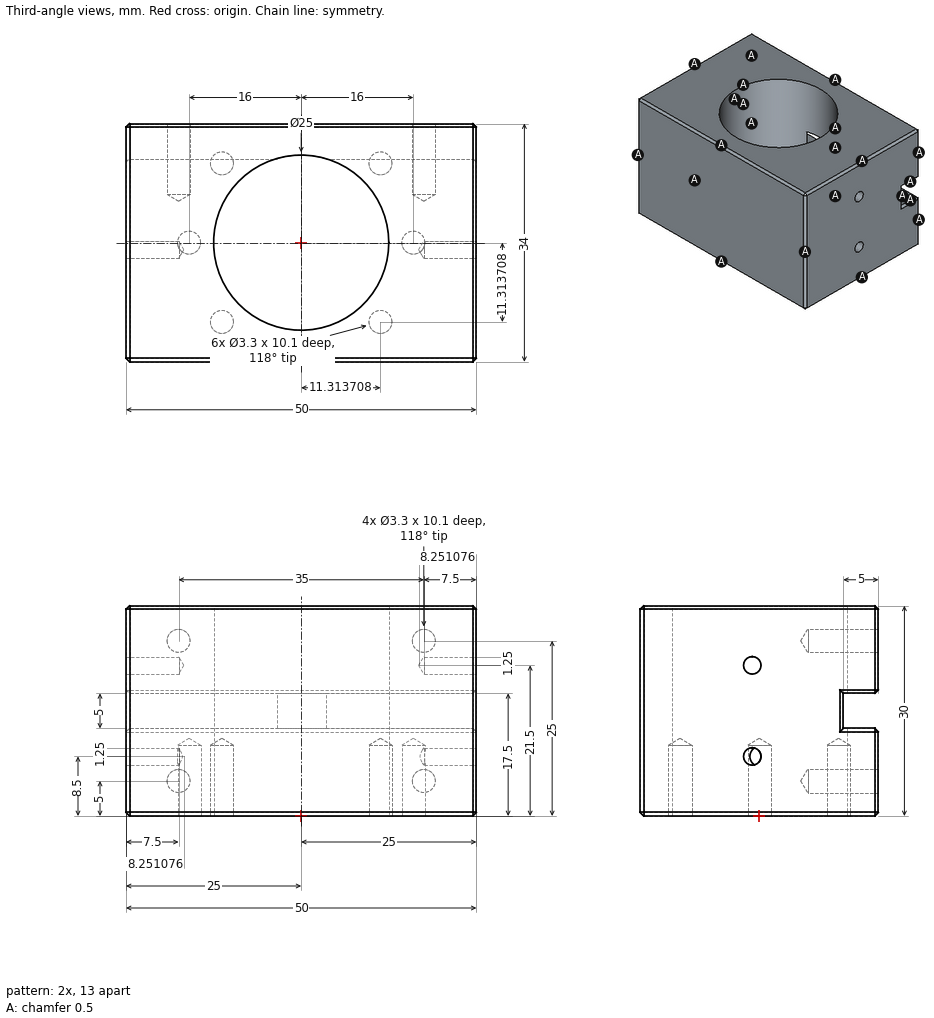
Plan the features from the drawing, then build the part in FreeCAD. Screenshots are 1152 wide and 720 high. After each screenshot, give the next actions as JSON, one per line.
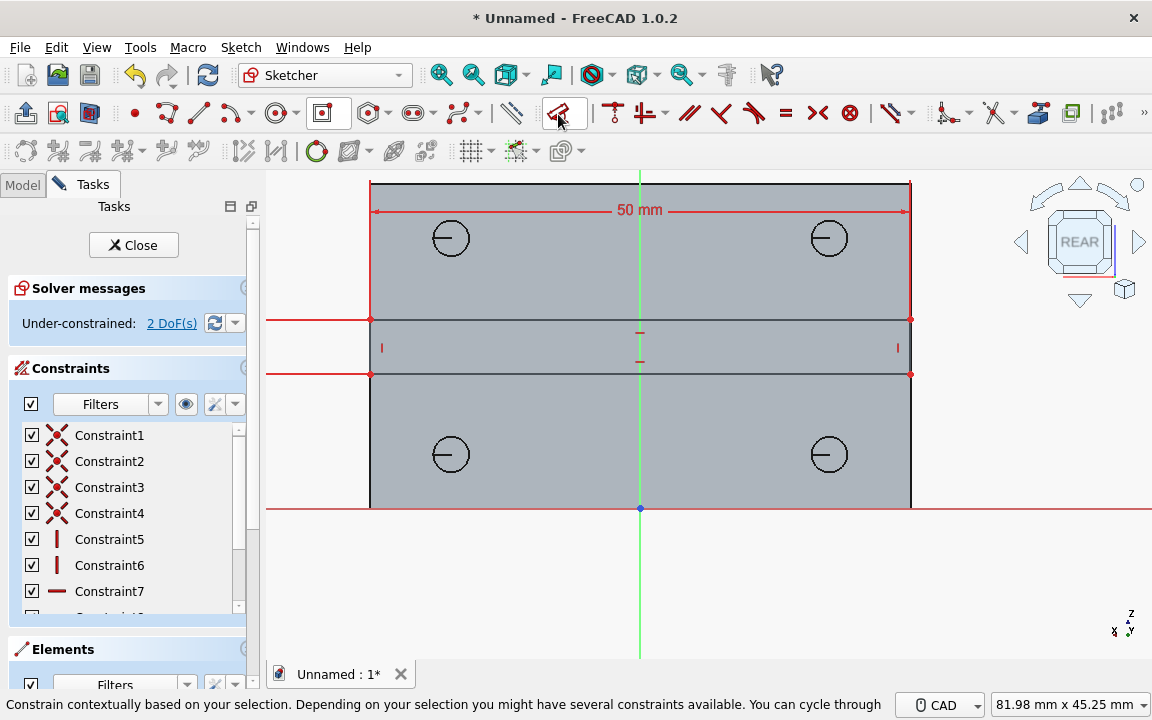
{"action": "left_click", "coordinate": [370, 320]}
{"action": "left_click", "coordinate": [505, 543]}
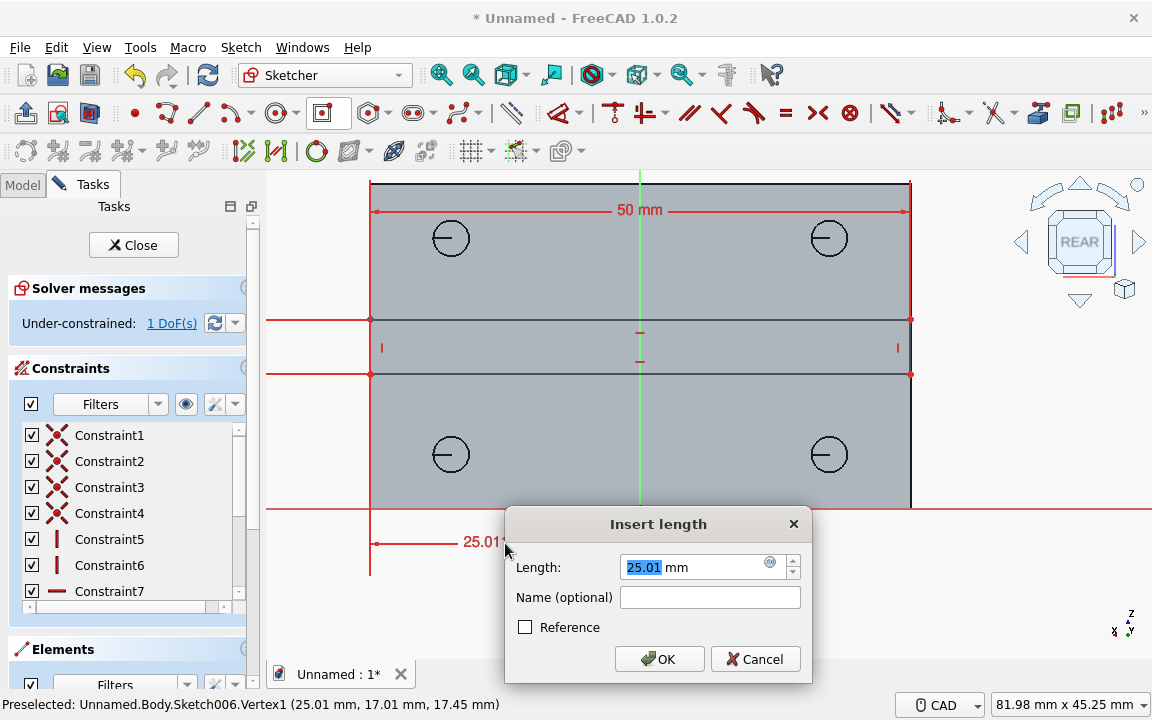
{"action": "type", "text": "25"}
{"action": "key", "text": "Return"}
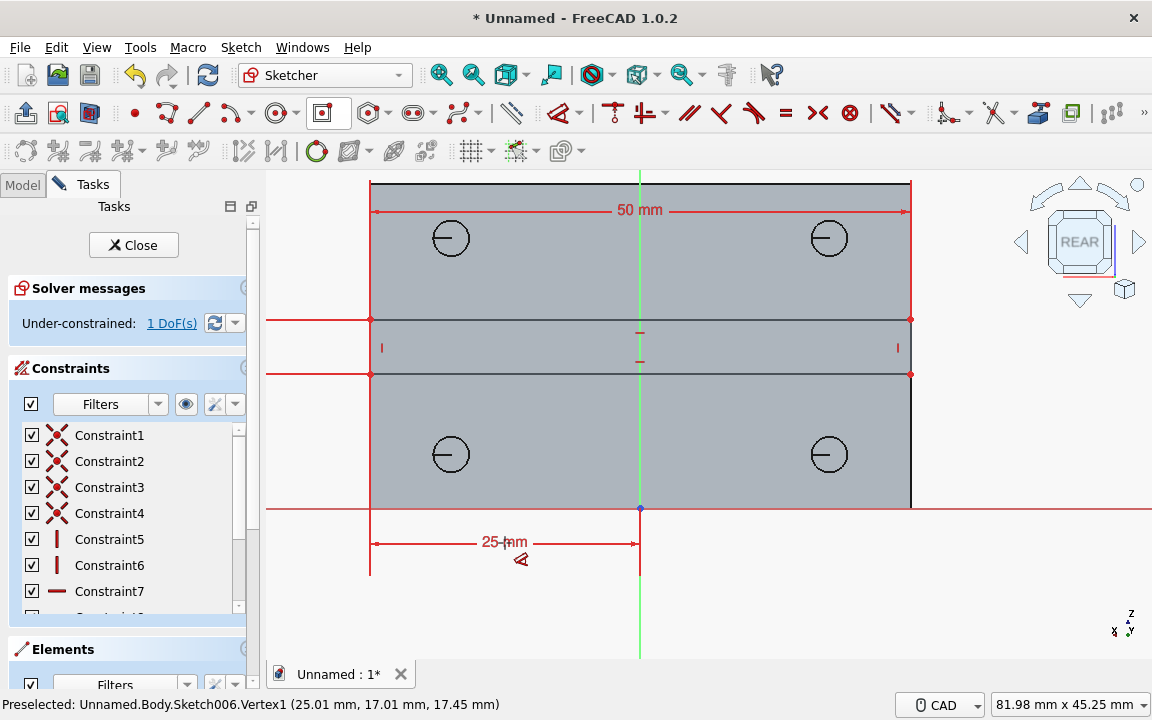
{"action": "left_click", "coordinate": [370, 320]}
{"action": "left_click", "coordinate": [336, 414]}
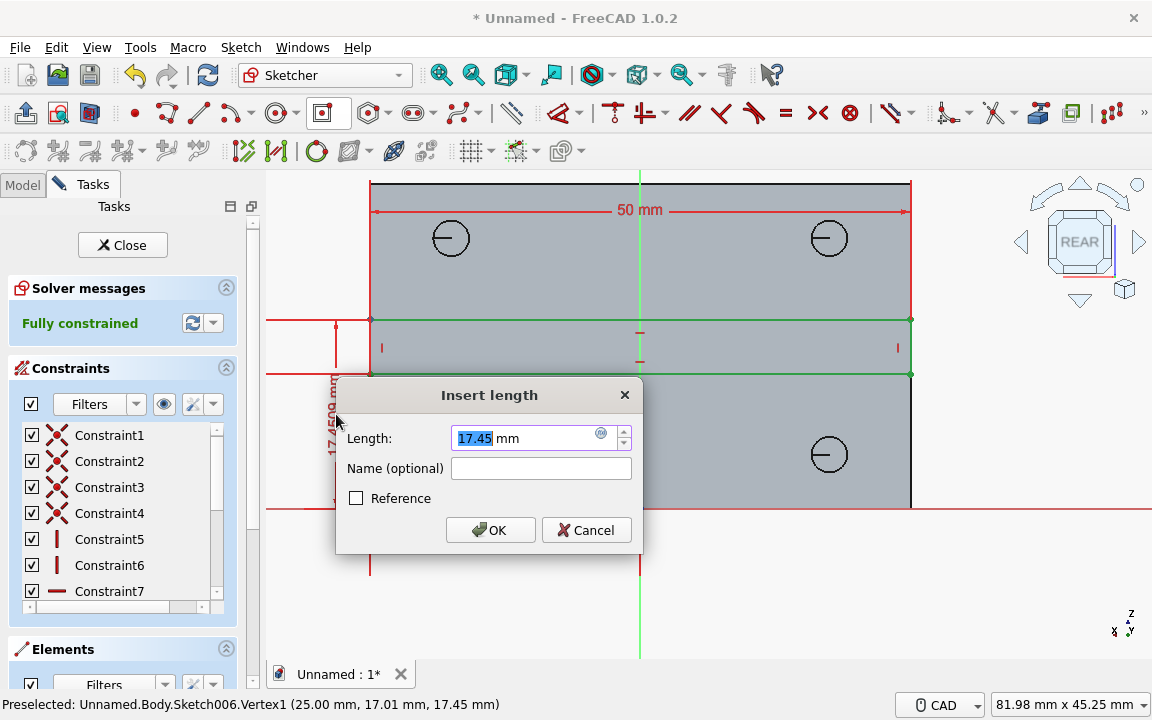
{"action": "type", "text": "17.5"}
{"action": "key", "text": "Return"}
{"action": "key", "text": "Escape"}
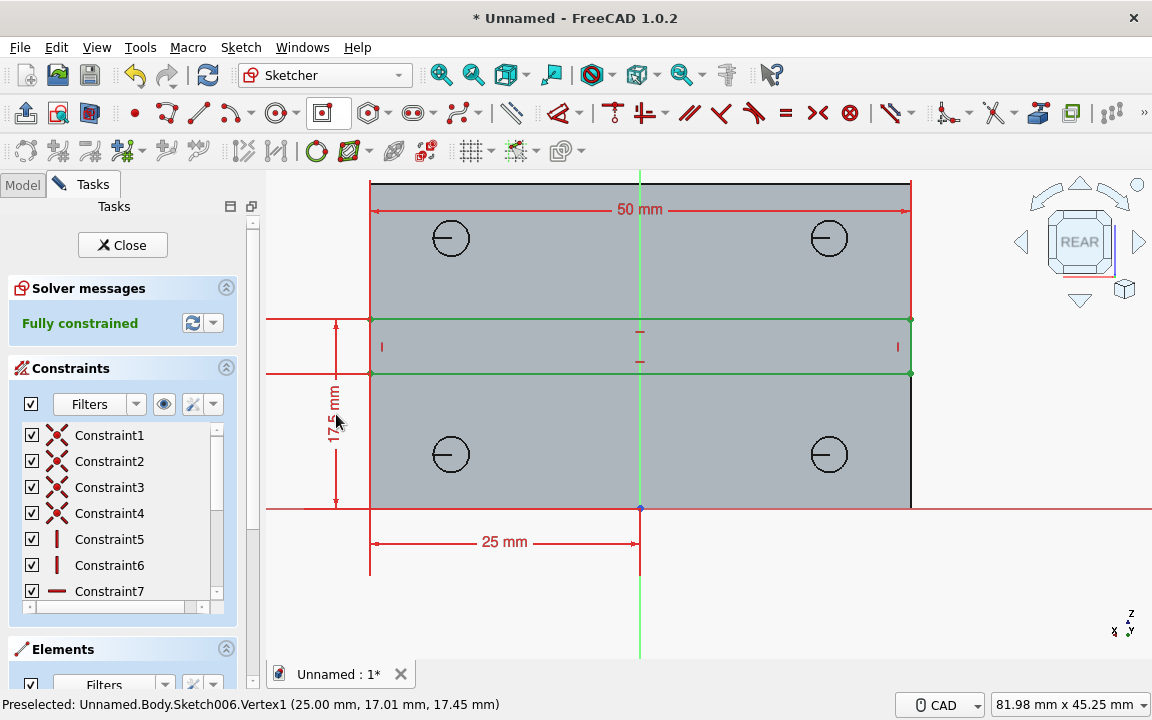
{"action": "left_click", "coordinate": [123, 245]}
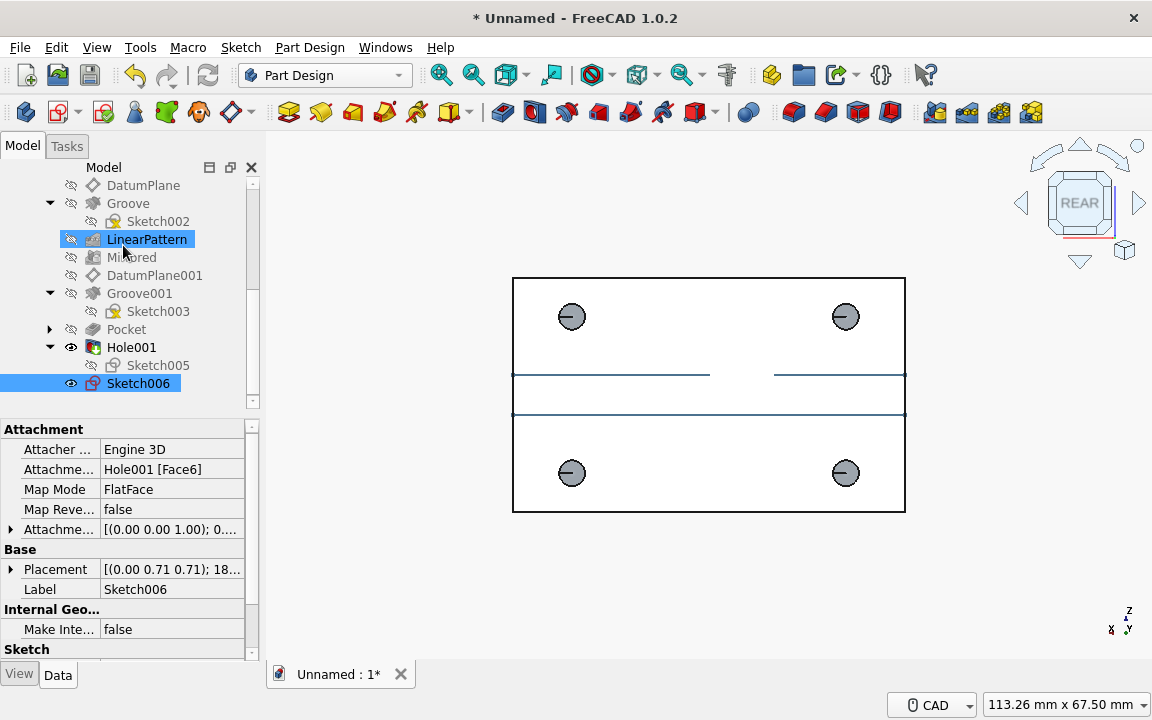
{"action": "left_click", "coordinate": [504, 112]}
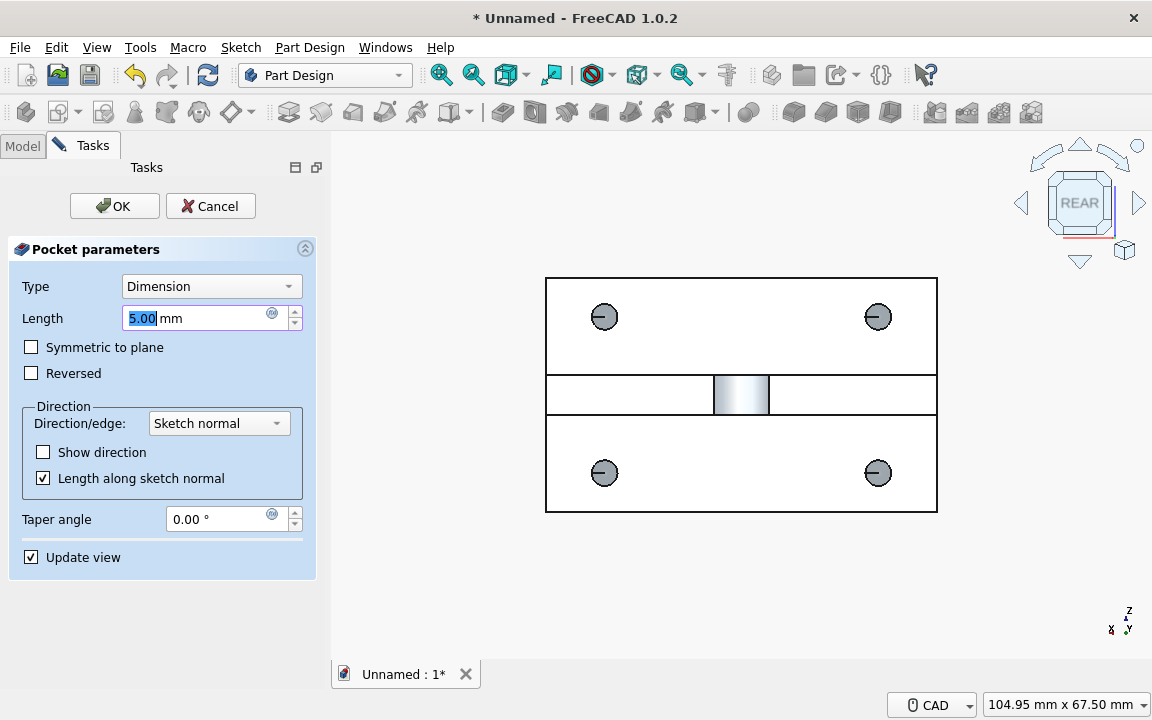
{"action": "type", "text": "5"}
{"action": "key", "text": "Tab"}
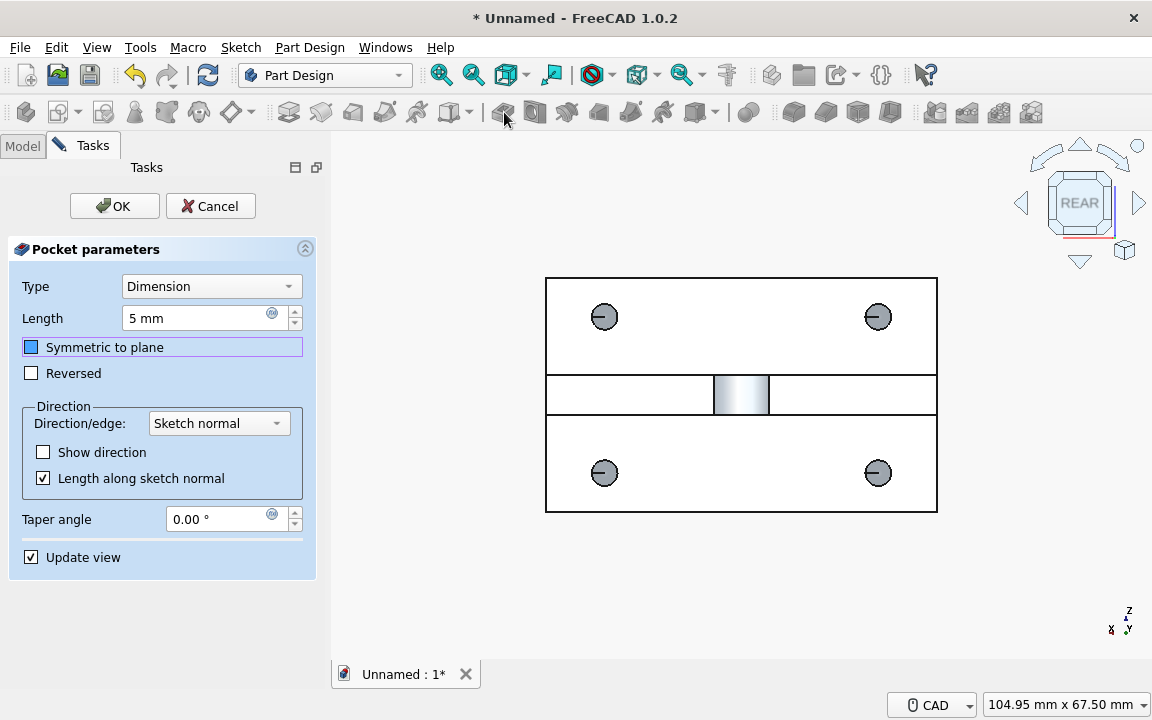
{"action": "left_click", "coordinate": [115, 206]}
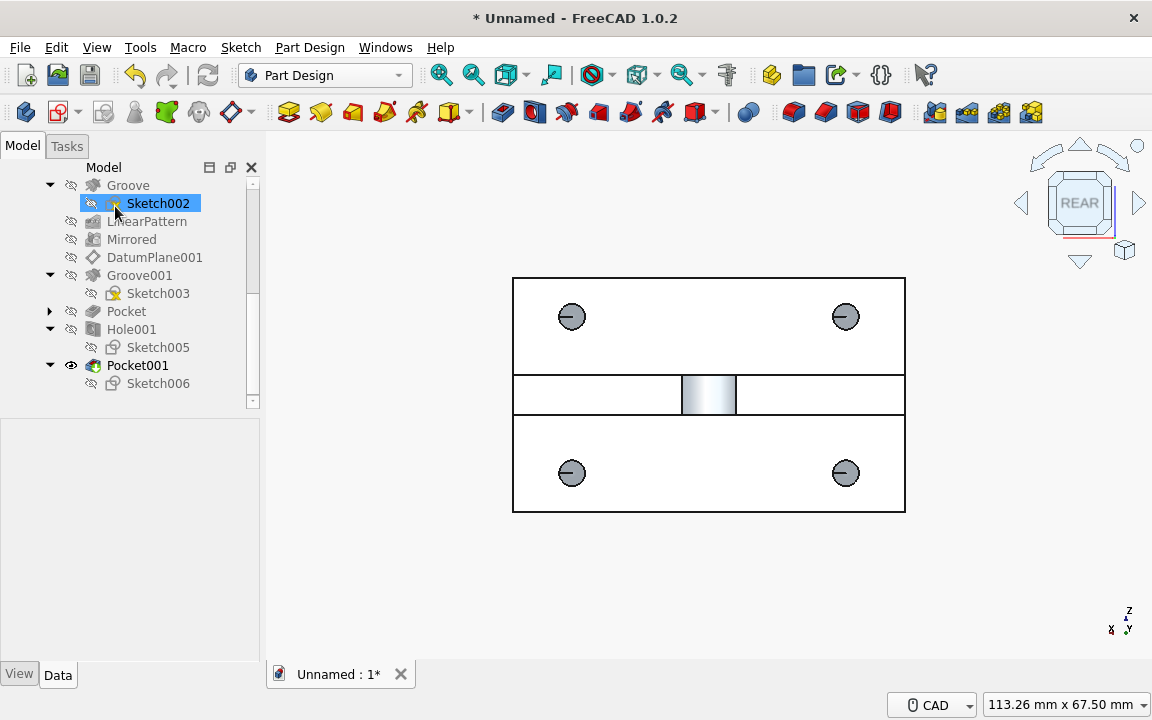
{"action": "key", "text": "v f"}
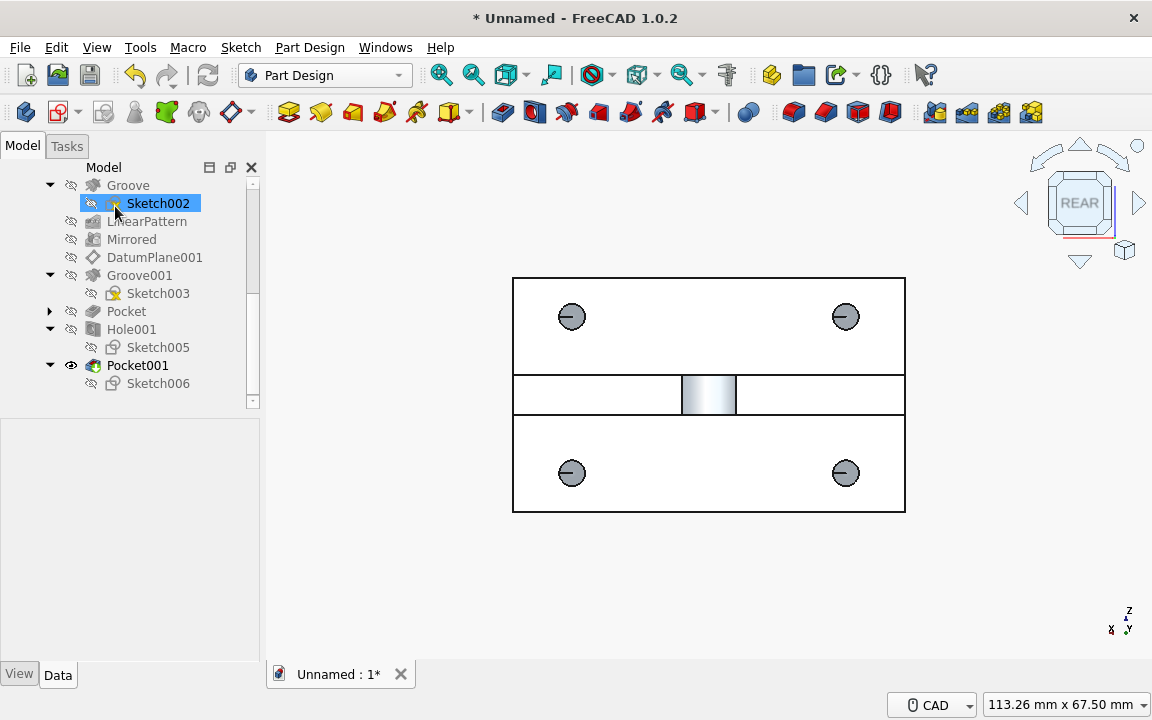
{"action": "left_click", "coordinate": [709, 374]}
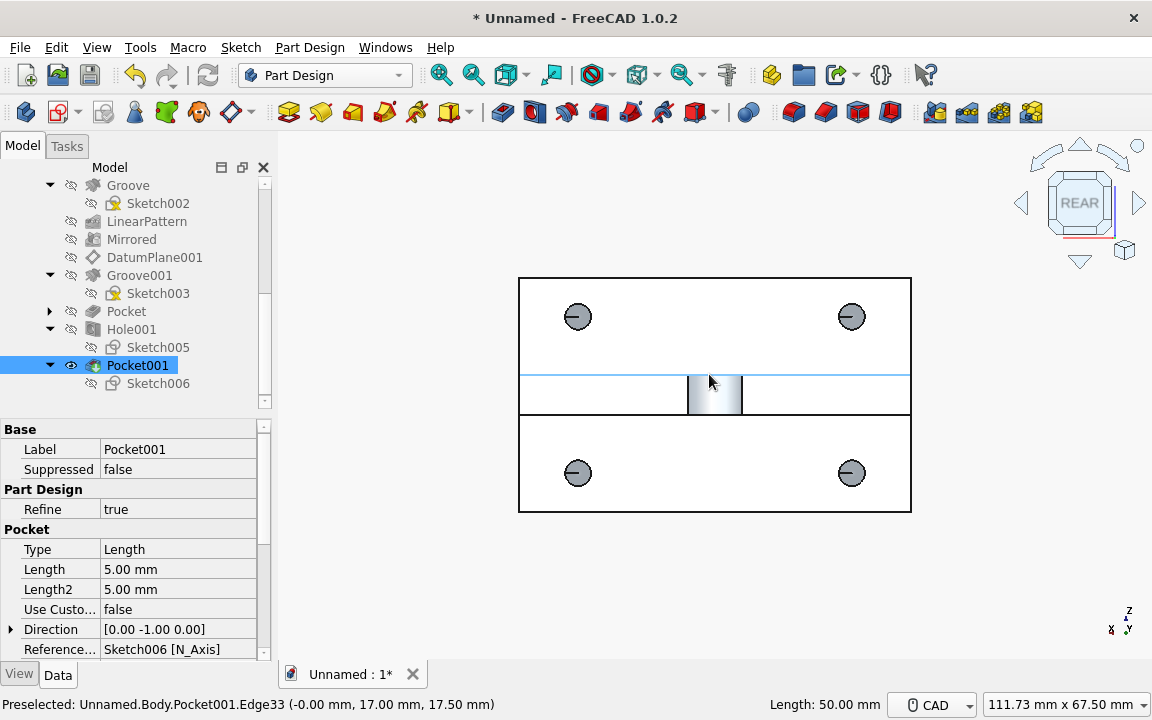
{"action": "left_click", "coordinate": [715, 511], "text": "ctrl"}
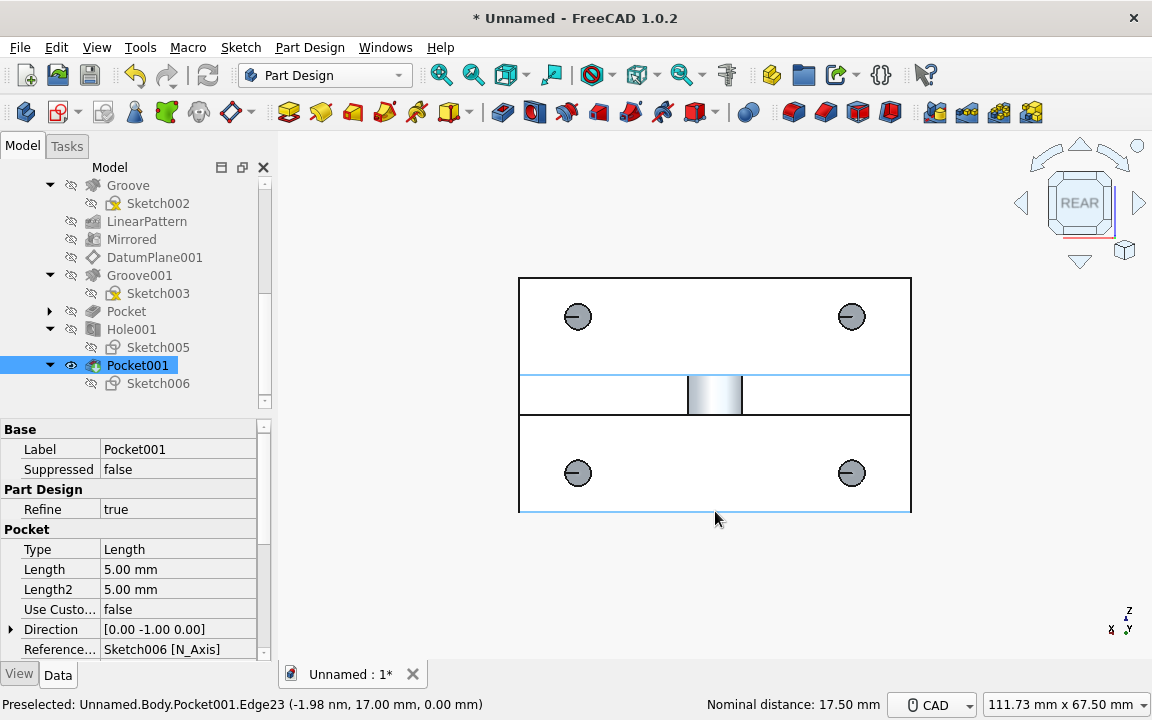
{"action": "left_click", "coordinate": [715, 277], "text": "ctrl"}